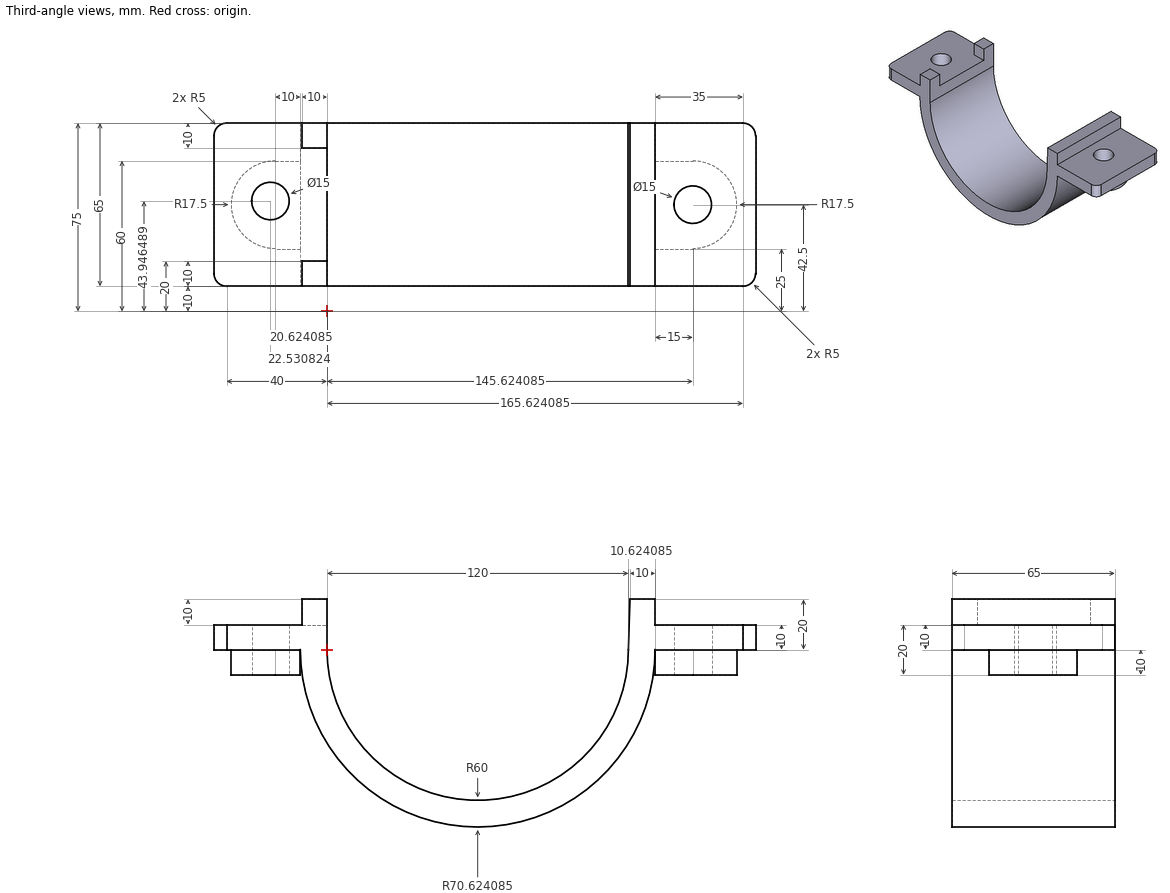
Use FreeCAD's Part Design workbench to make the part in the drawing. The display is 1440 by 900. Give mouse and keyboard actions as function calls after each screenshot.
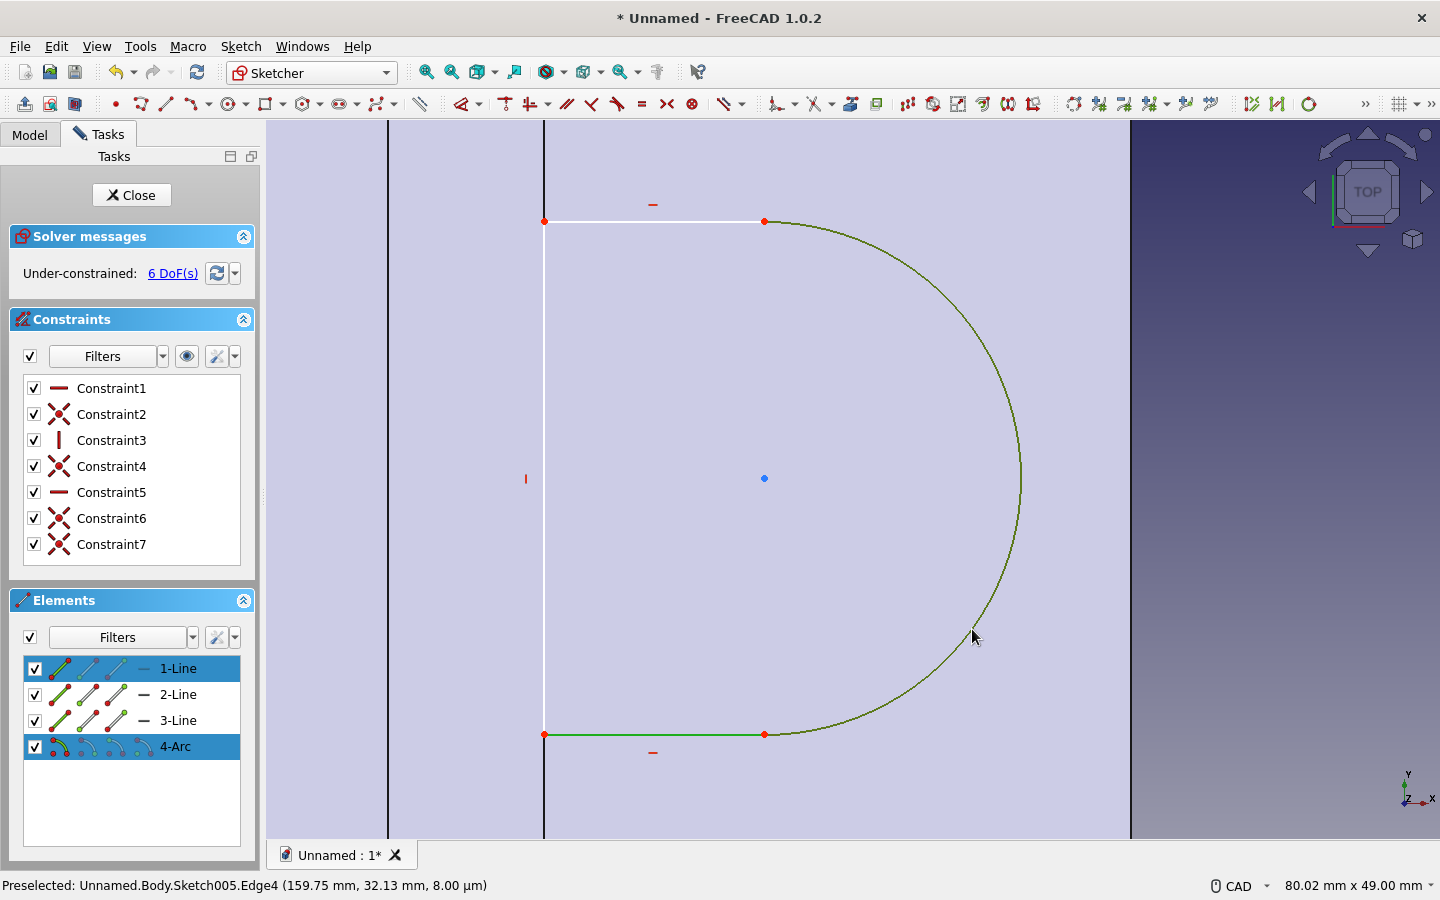
click(617, 104)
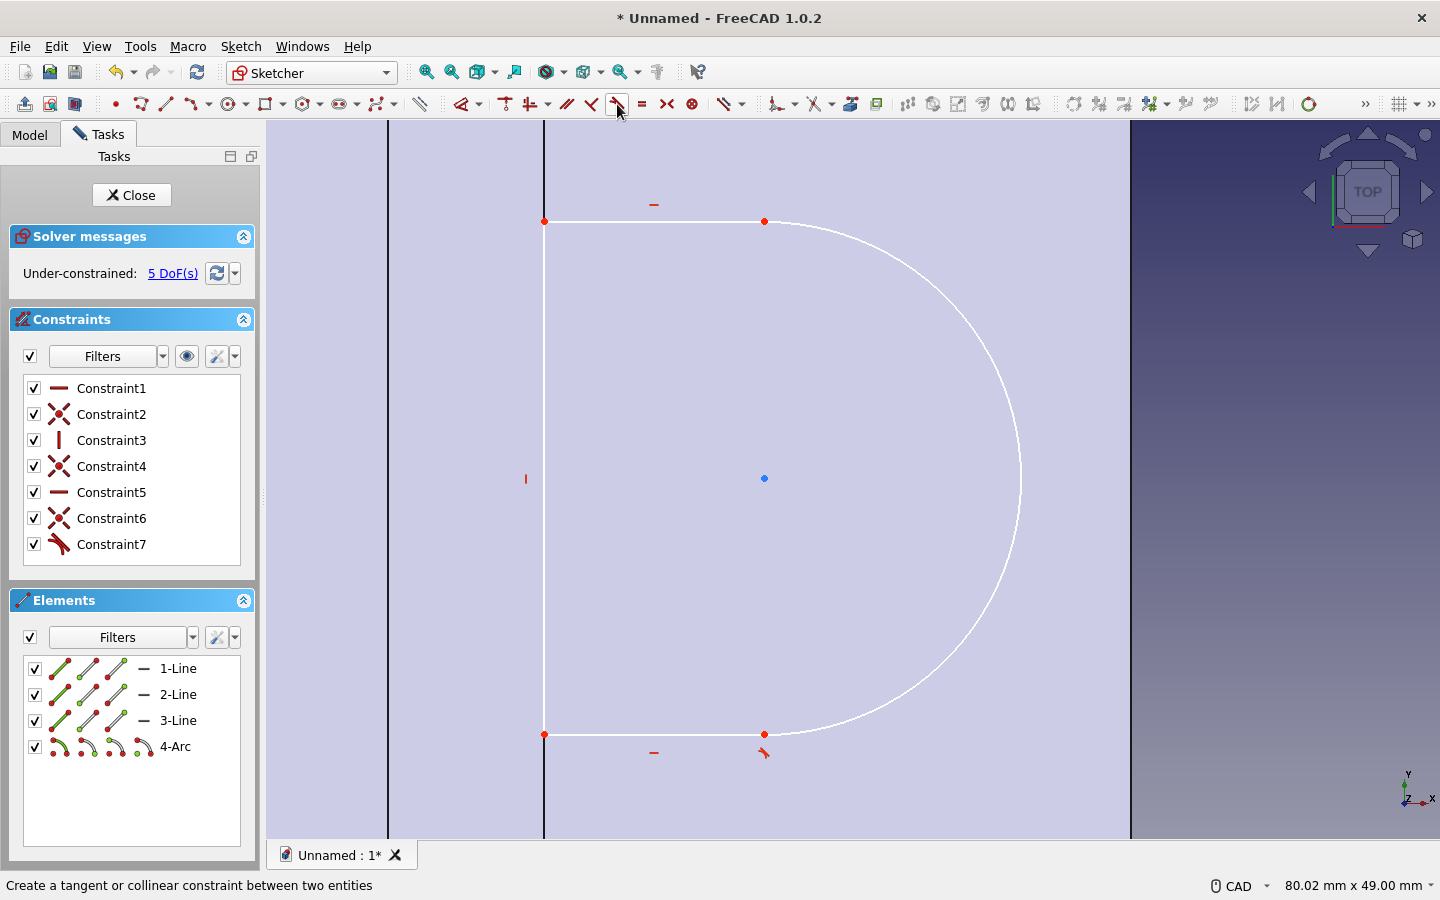
click(610, 222)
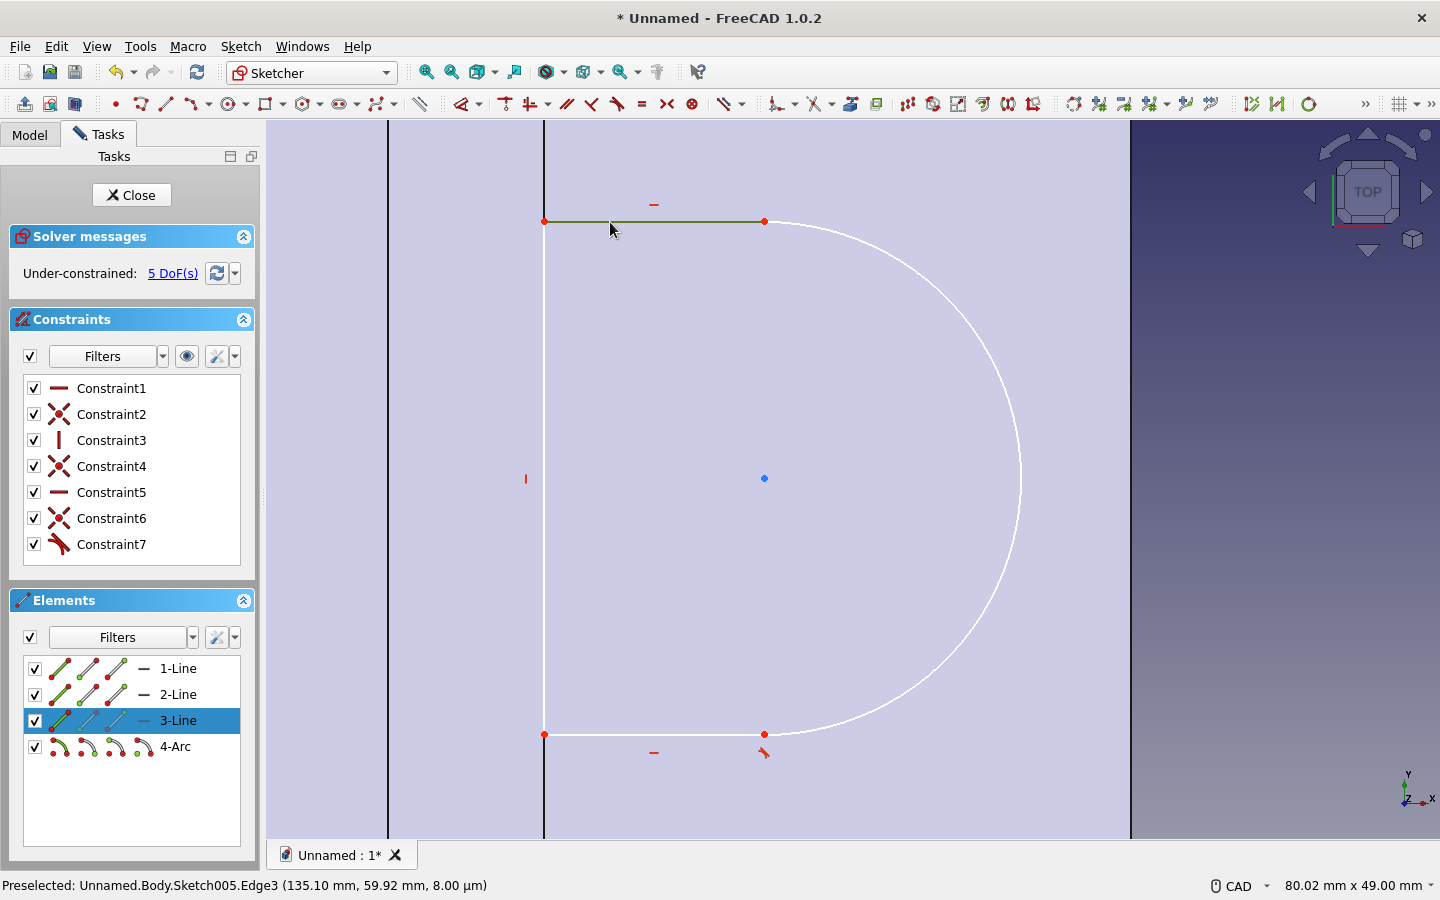
click(972, 629)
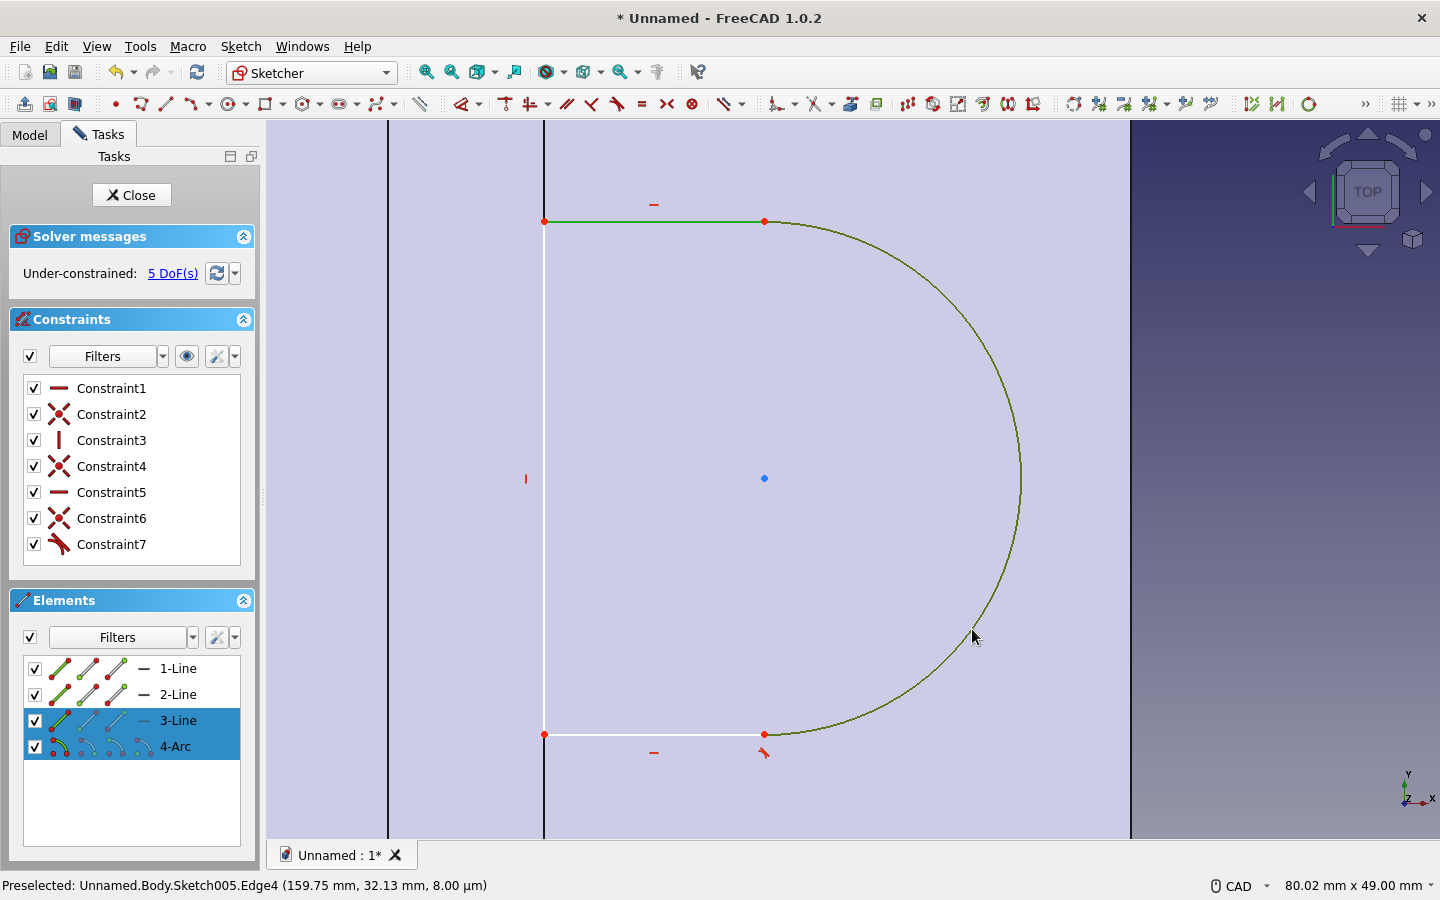
key(t)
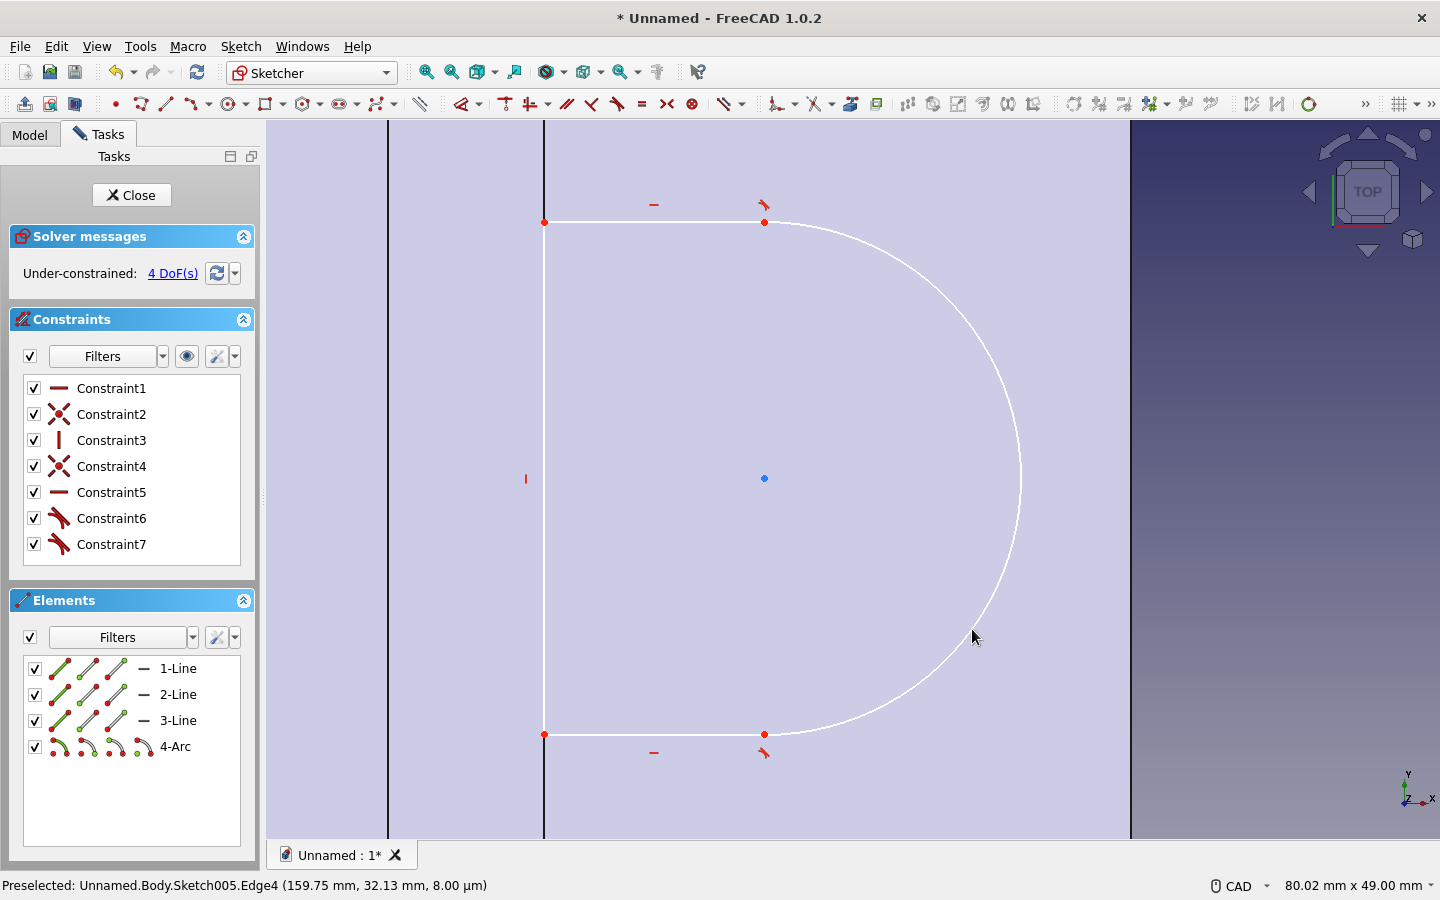
key(d)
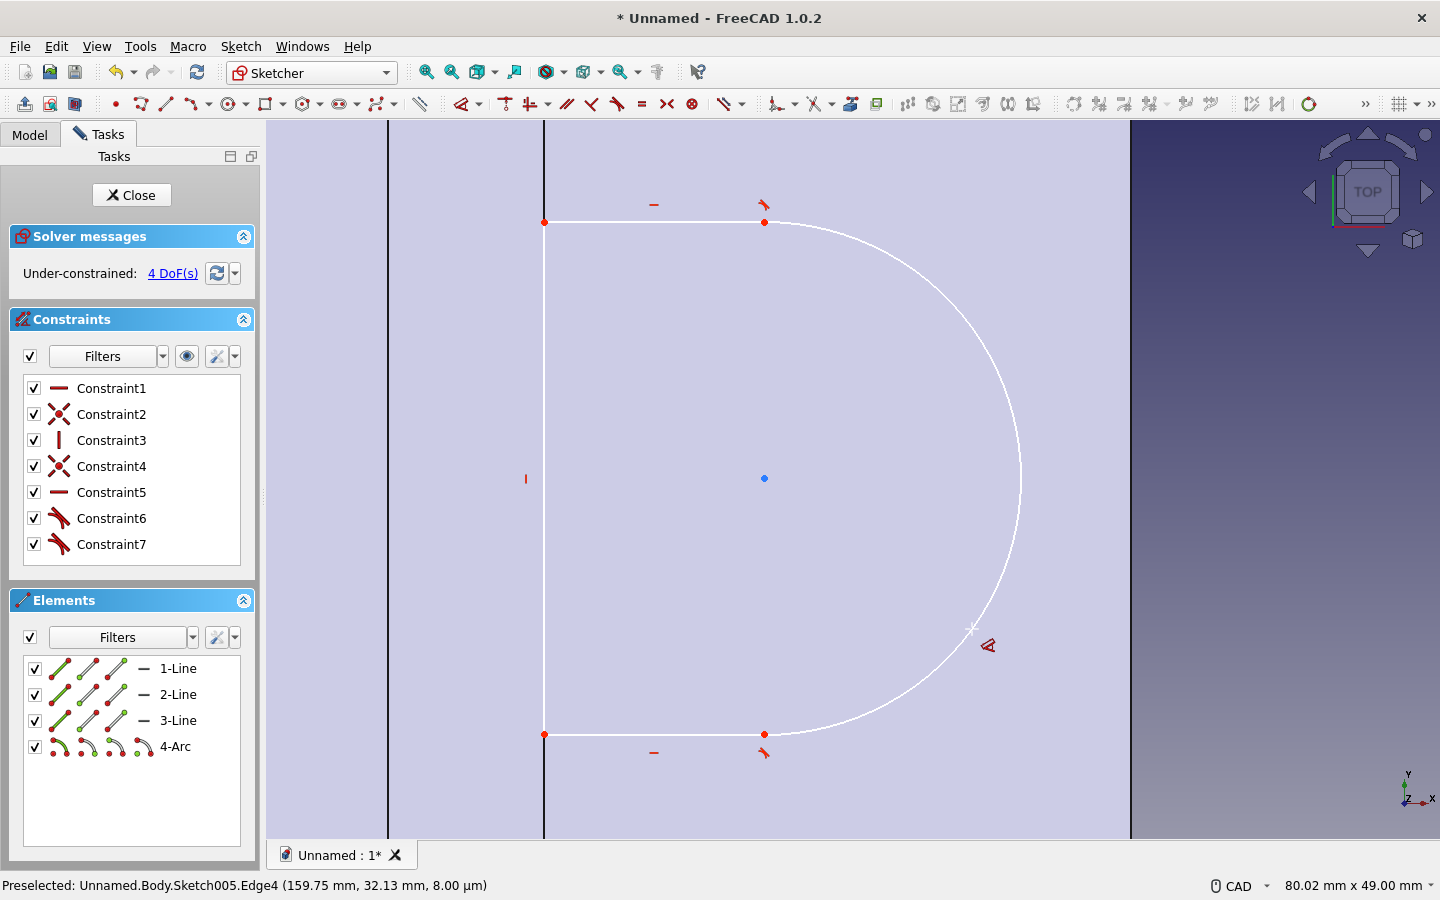
click(972, 629)
click(998, 648)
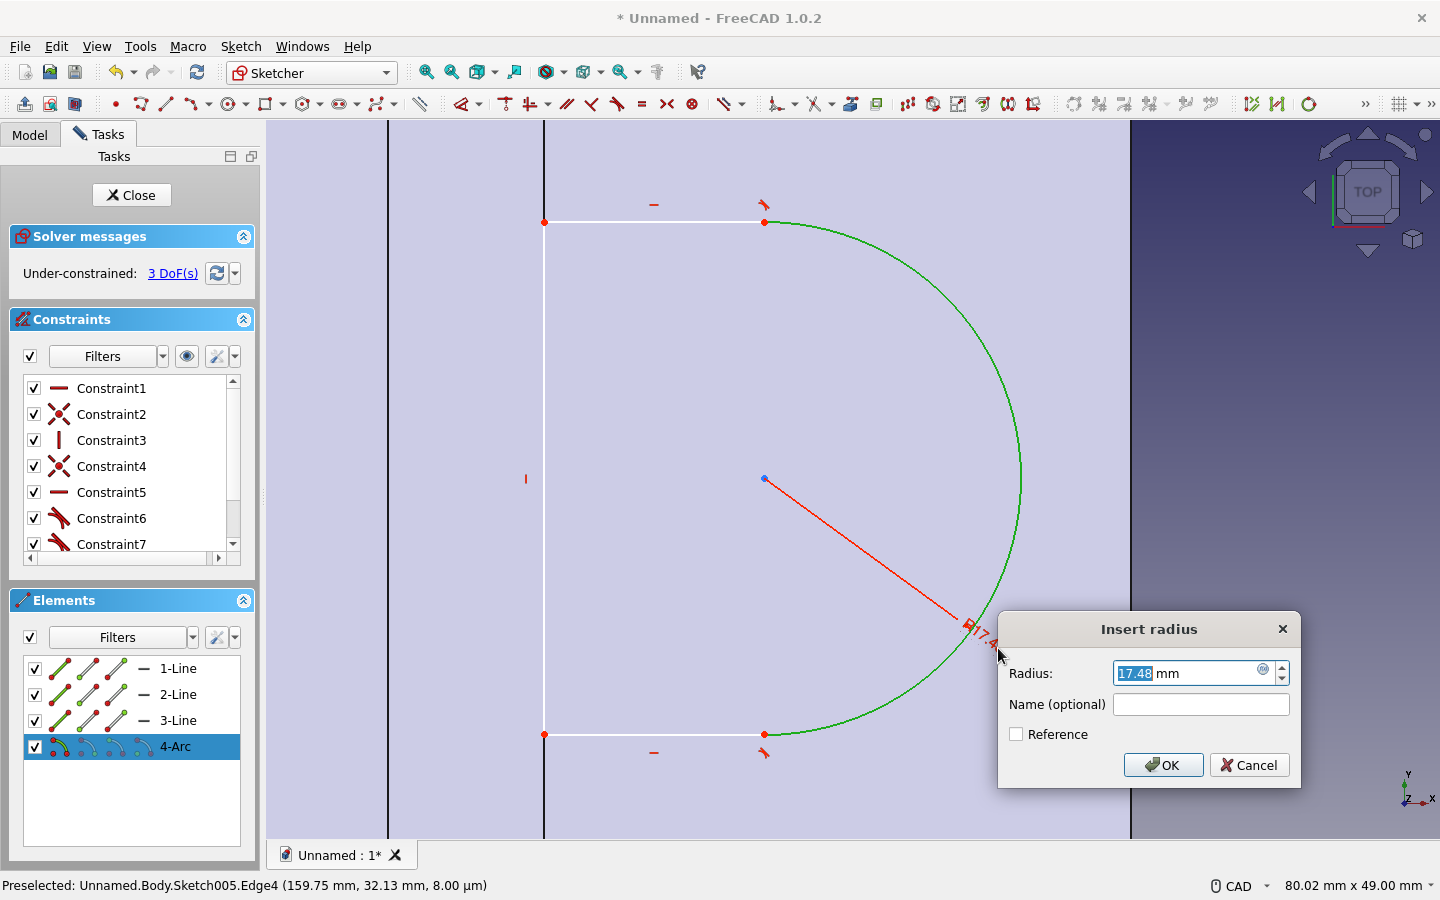
text(17.5)
key(Return)